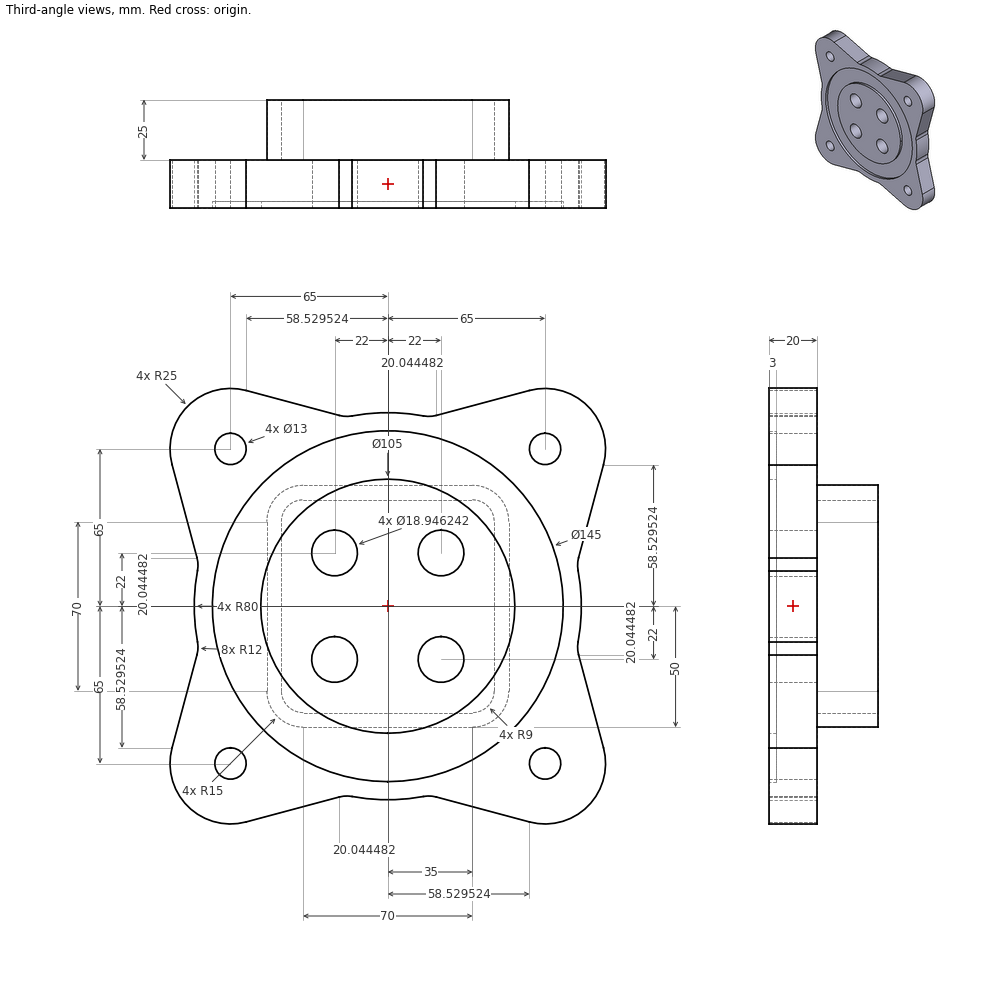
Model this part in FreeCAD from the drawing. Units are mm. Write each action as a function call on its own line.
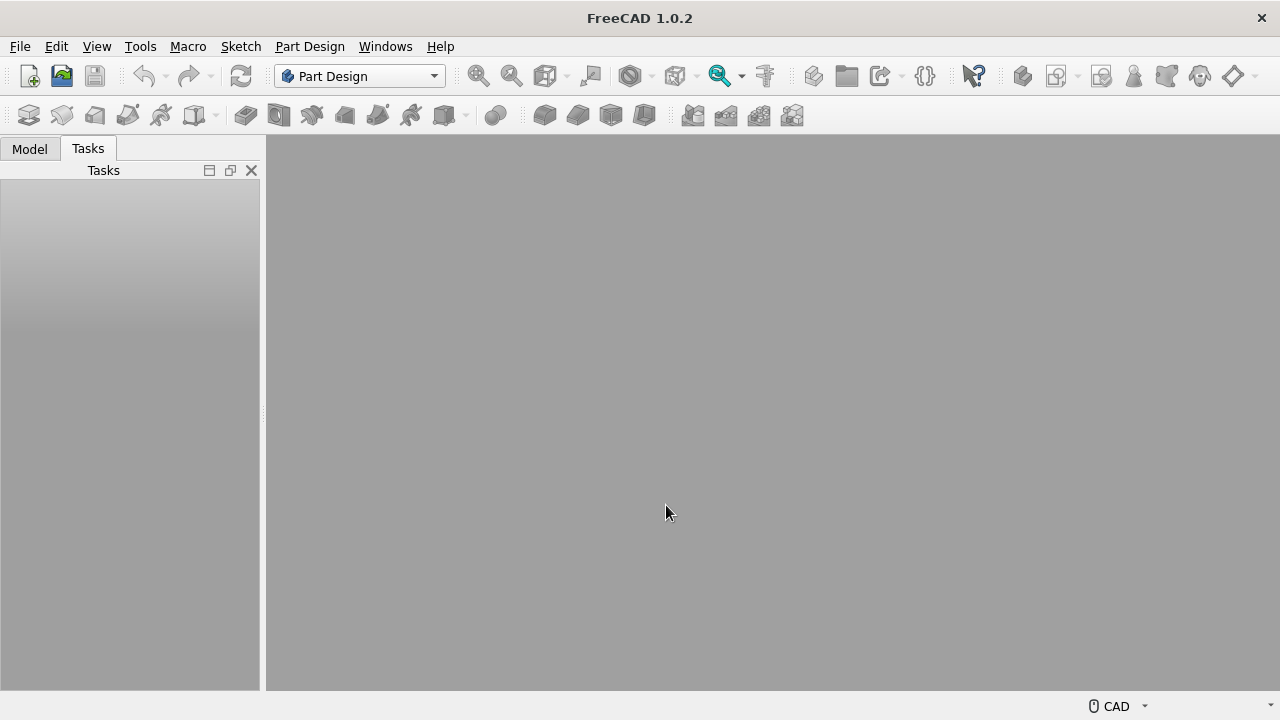
click(29, 76)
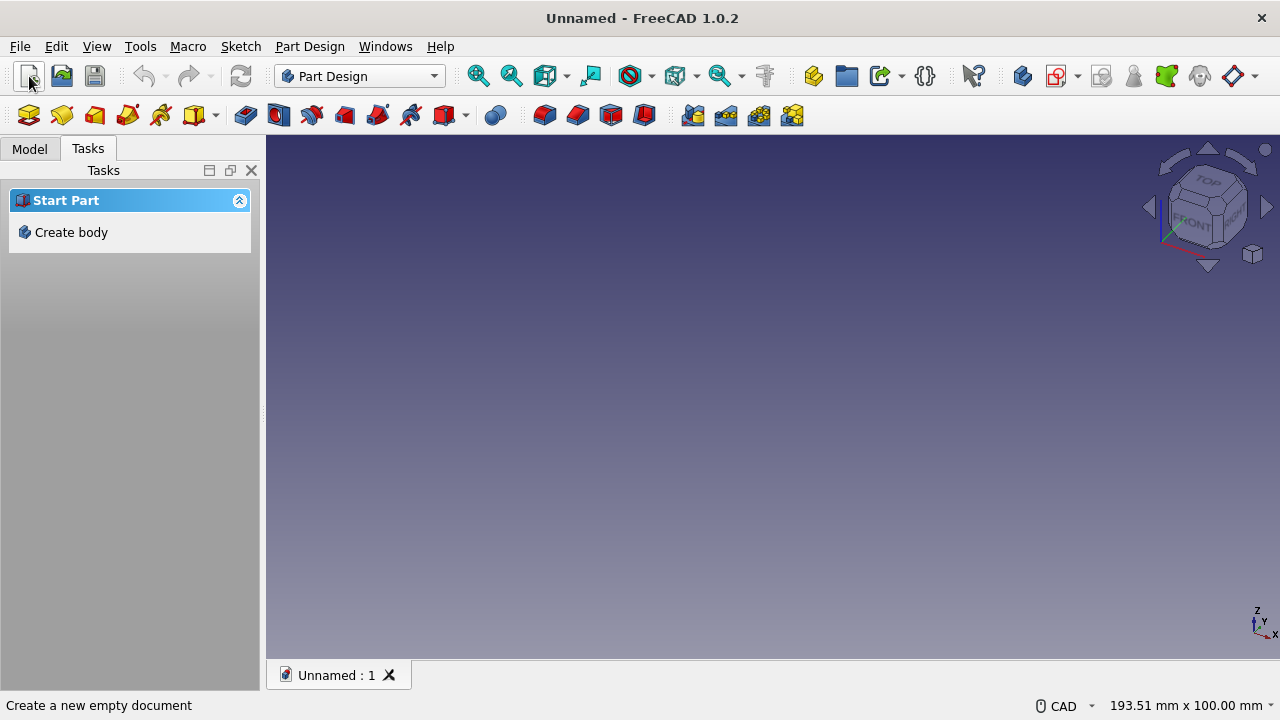
click(1056, 76)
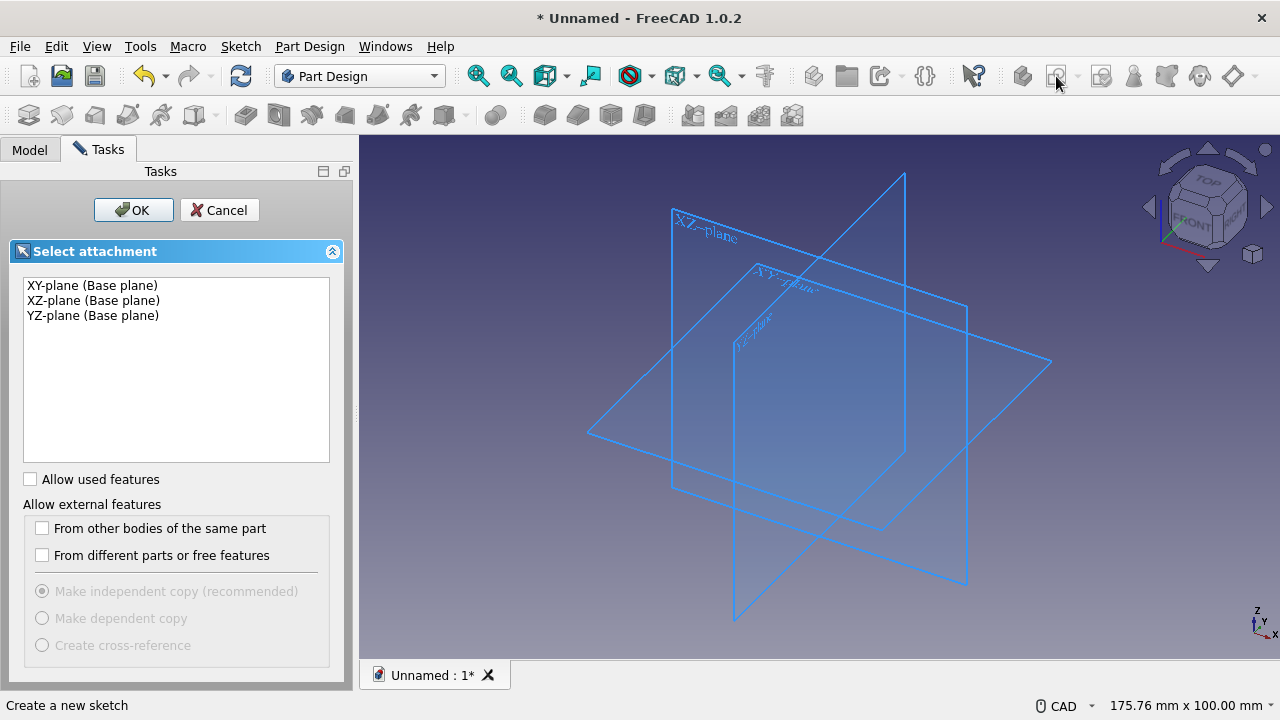
click(84, 300)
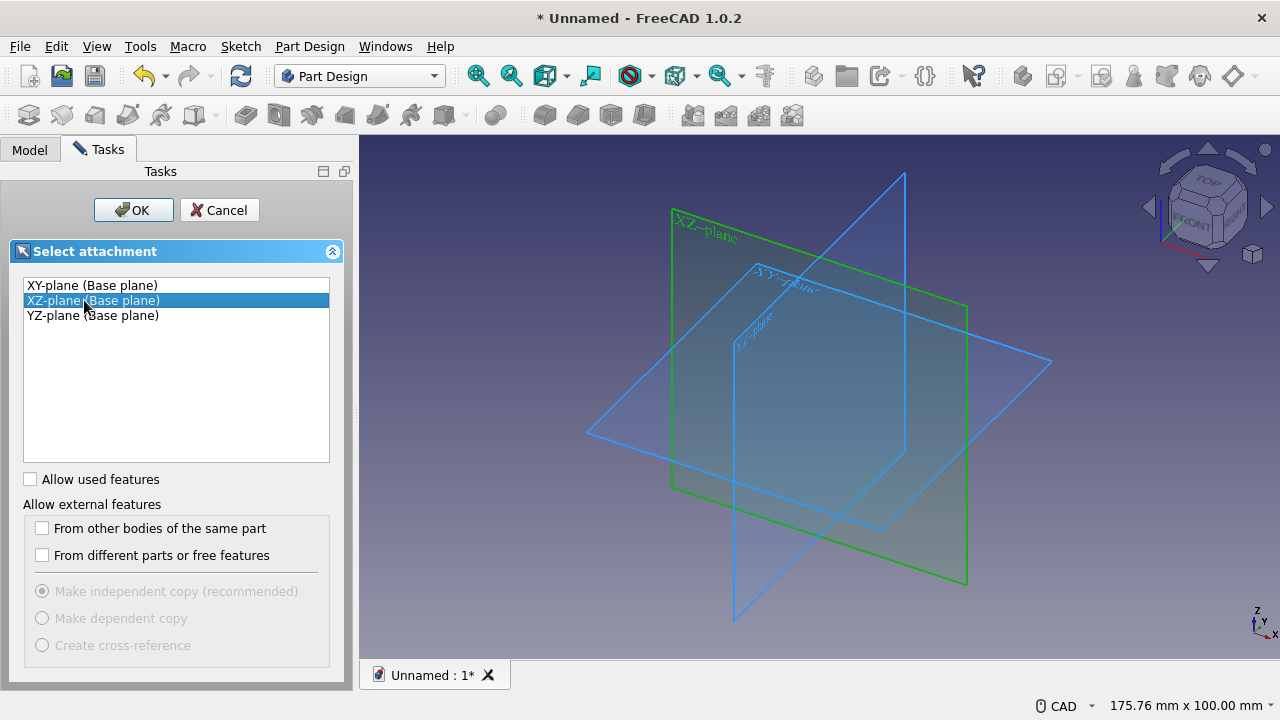
click(134, 210)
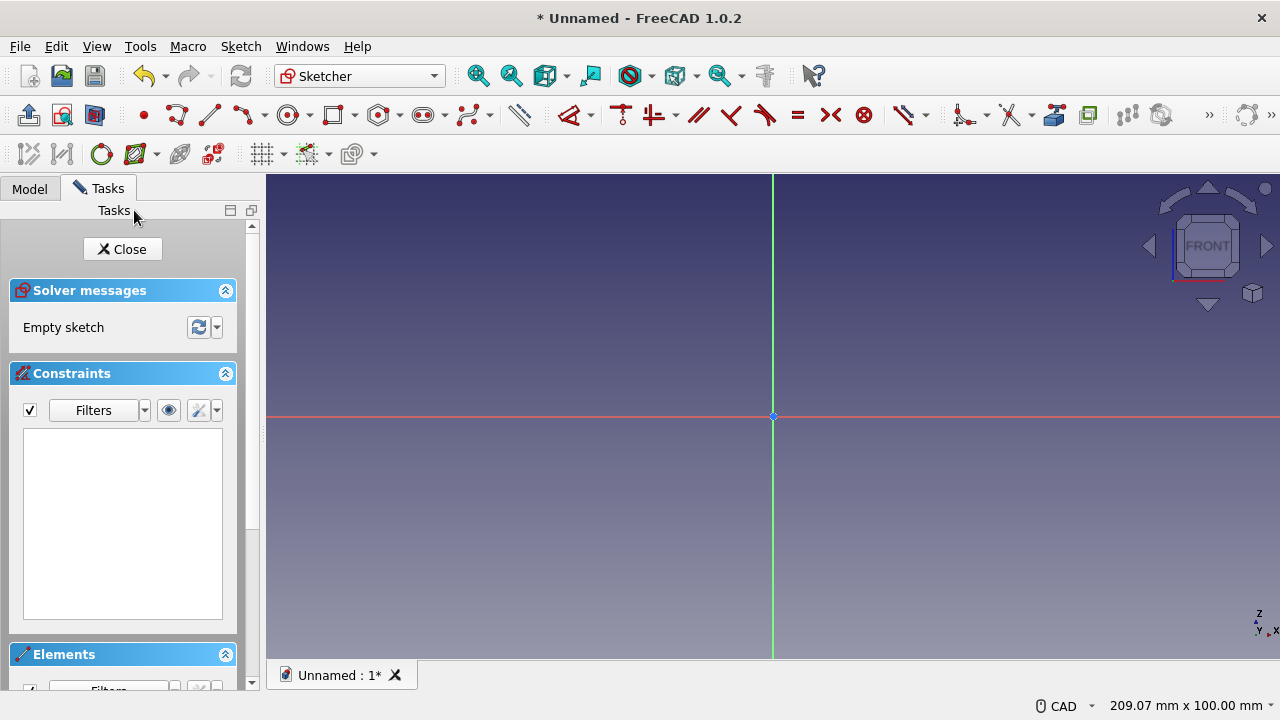
scroll(665, 417, down, 5)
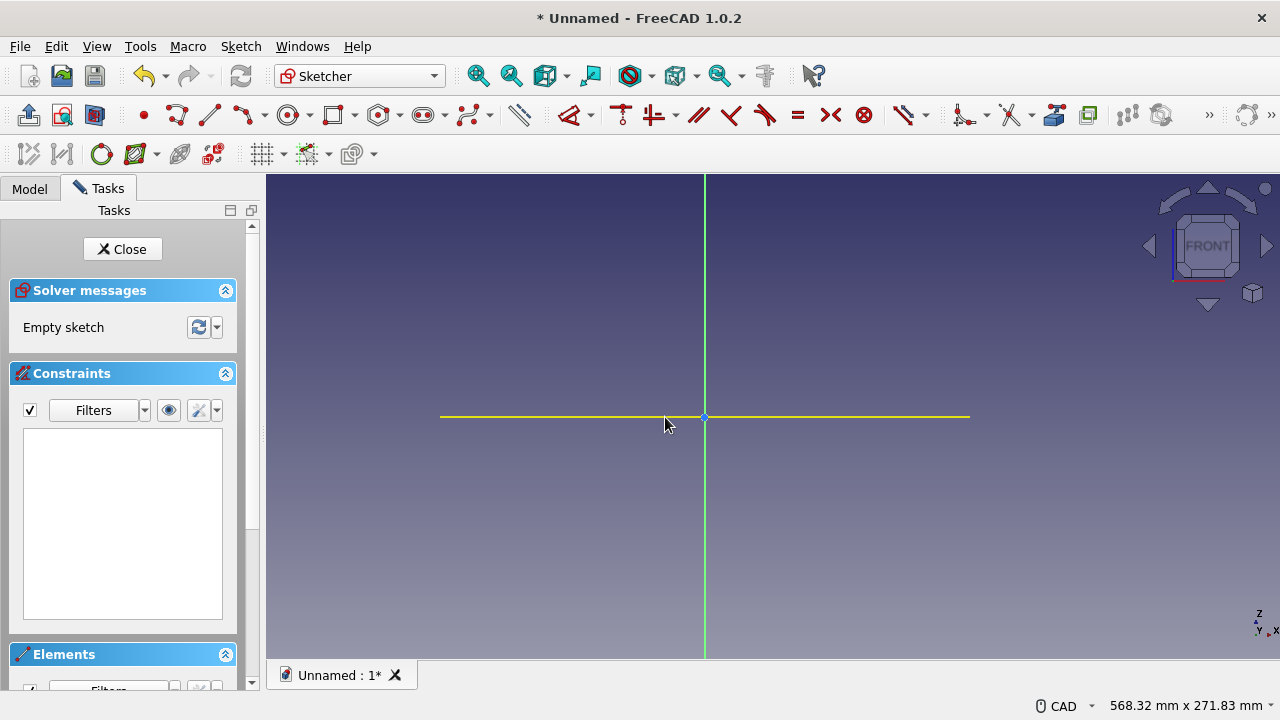
click(210, 116)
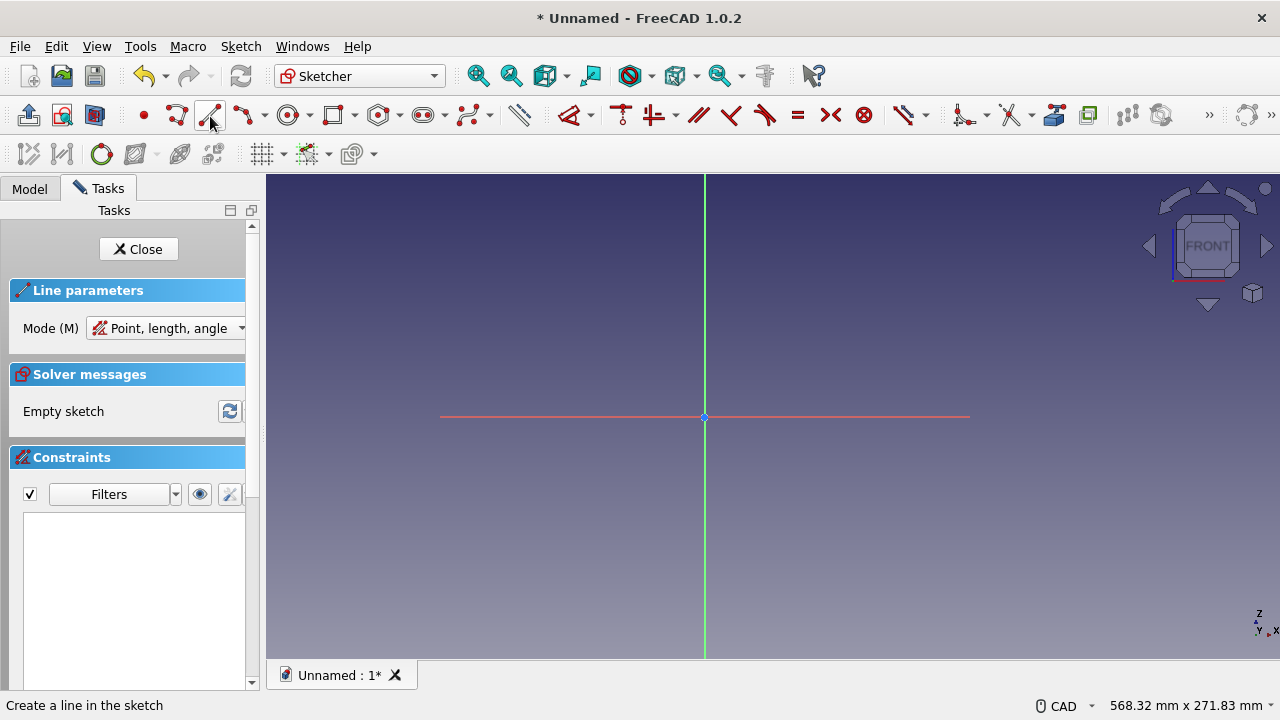
click(546, 522)
click(564, 453)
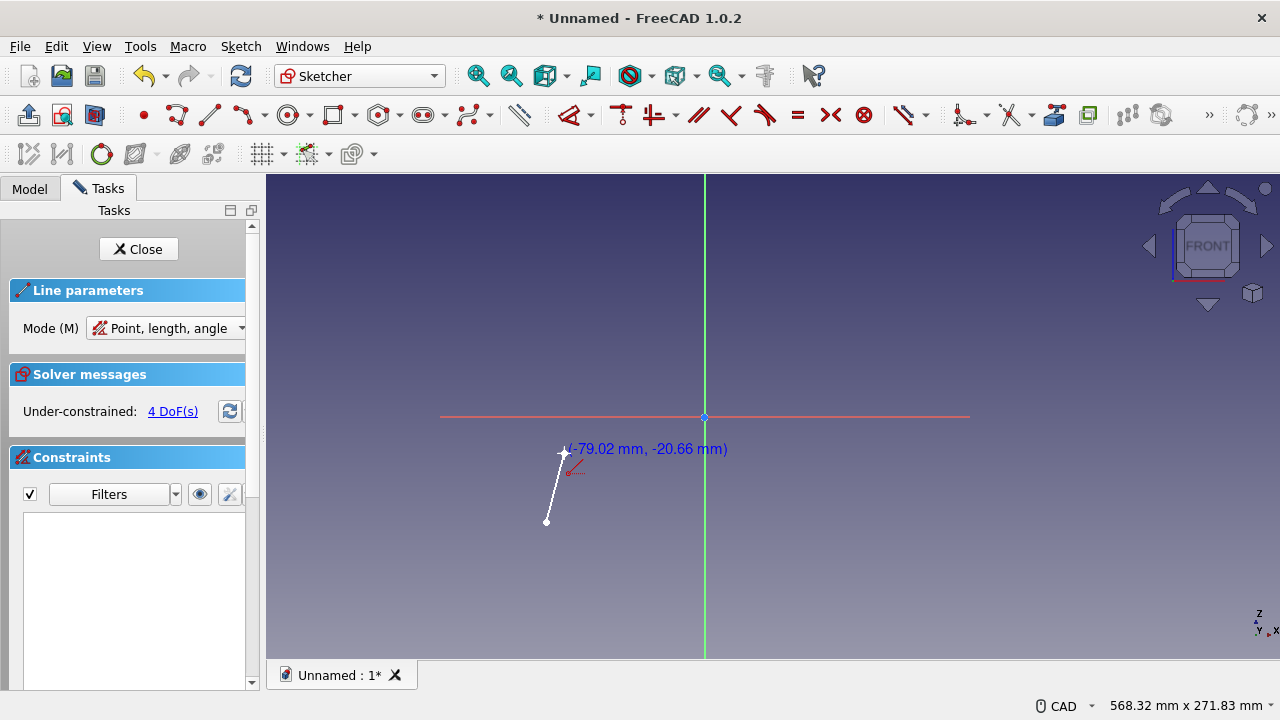
click(564, 381)
click(546, 313)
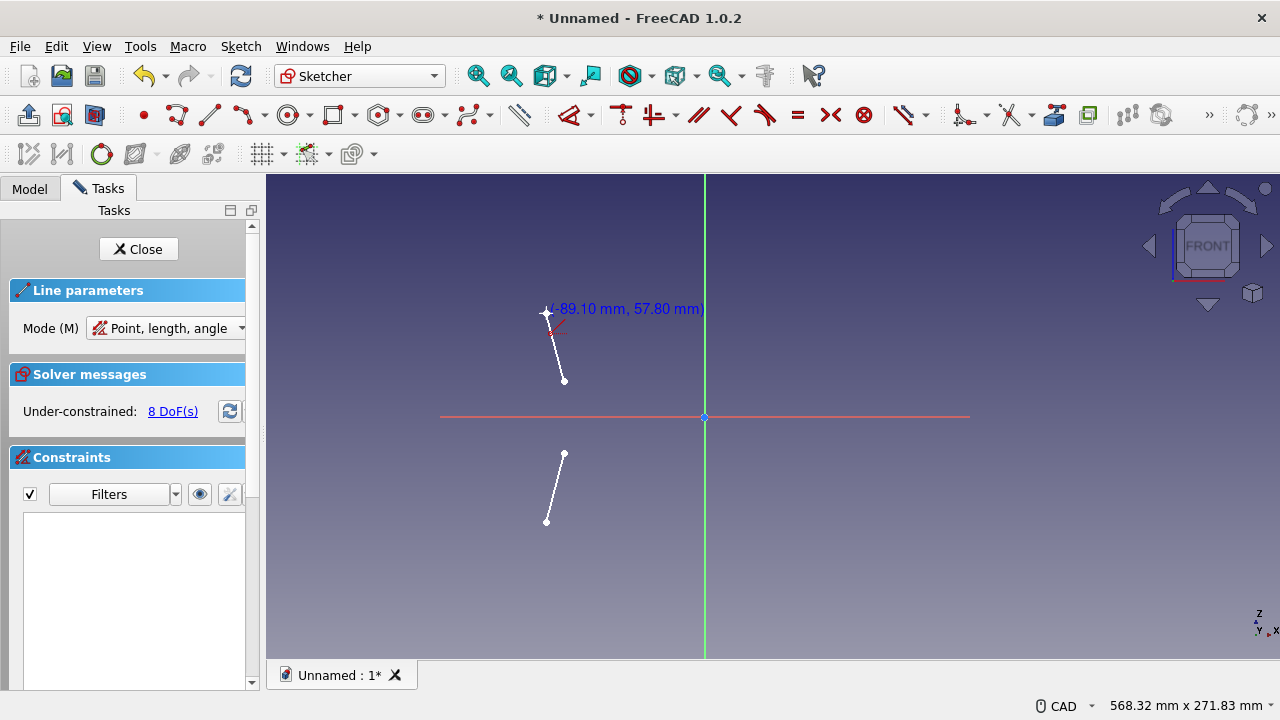
click(601, 258)
click(669, 276)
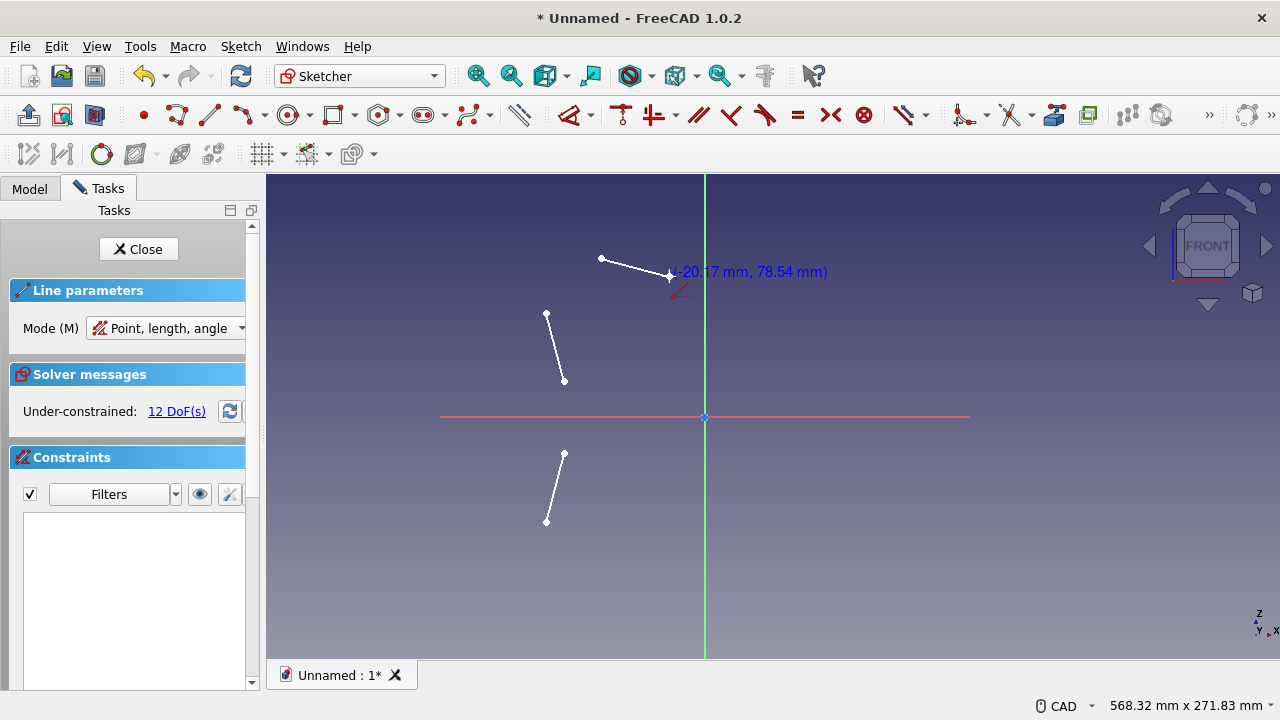
click(741, 276)
click(809, 258)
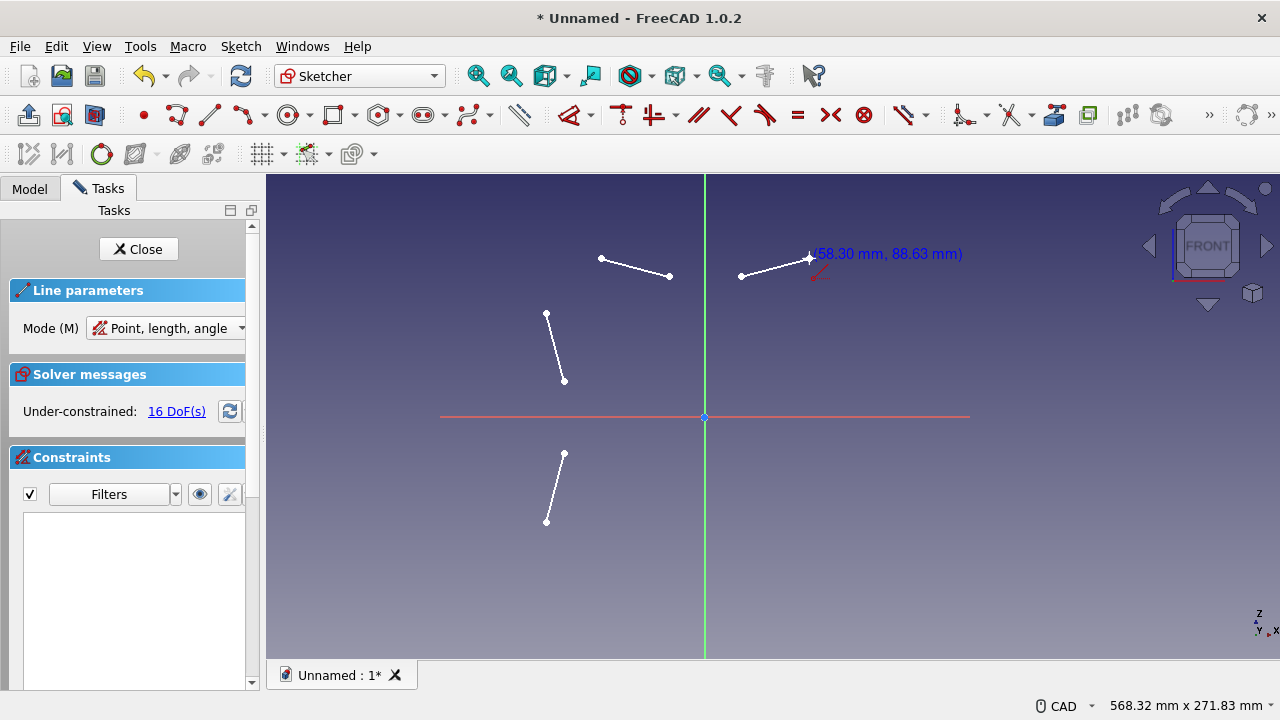
click(864, 313)
click(846, 381)